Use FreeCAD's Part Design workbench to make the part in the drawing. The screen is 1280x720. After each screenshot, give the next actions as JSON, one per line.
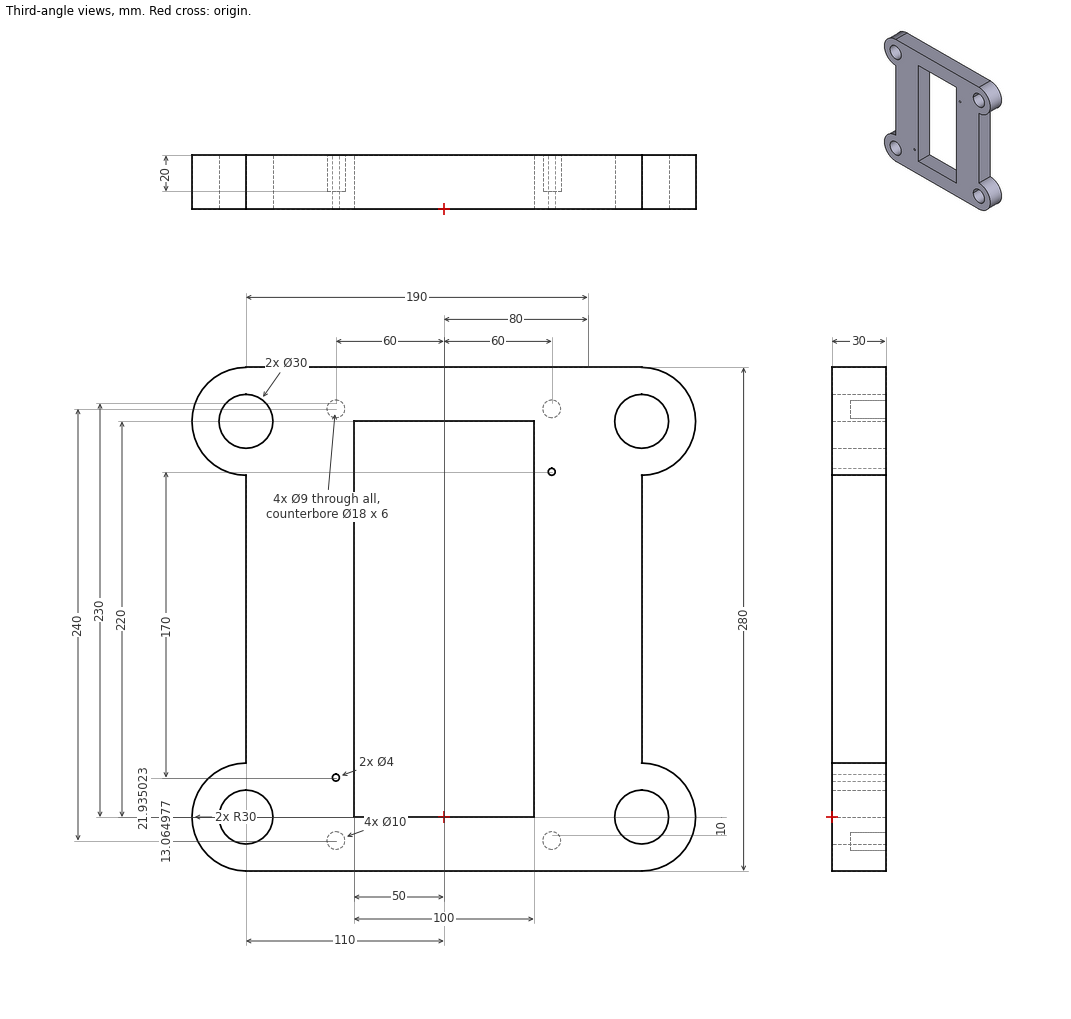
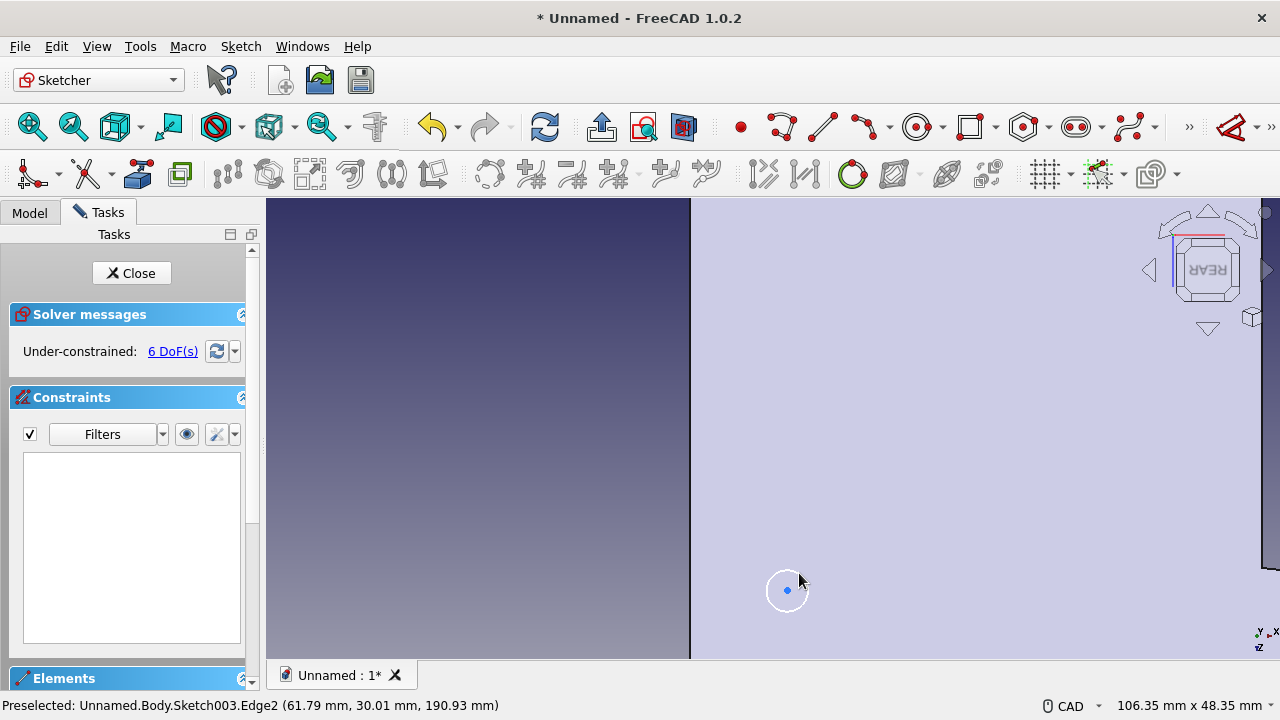
{"action": "scroll", "coordinate": [802, 577], "scroll_direction": "down", "scroll_amount": 9}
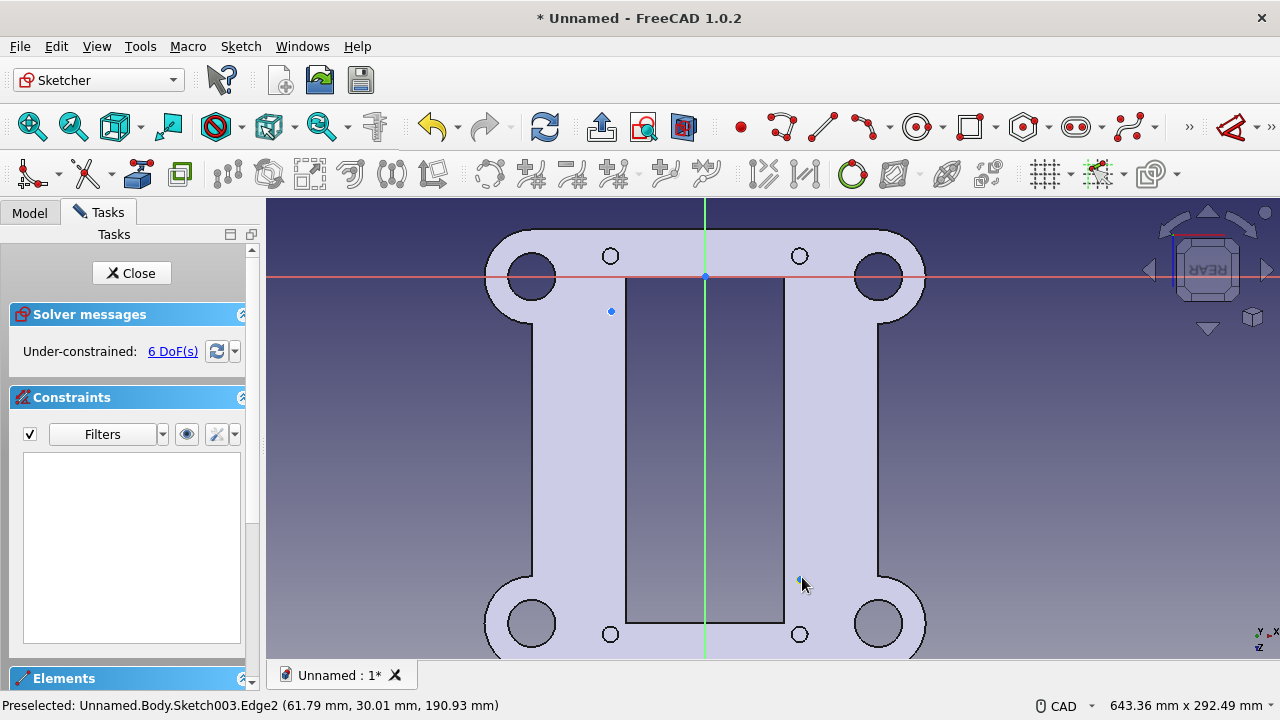
{"action": "scroll", "coordinate": [613, 310], "scroll_direction": "up", "scroll_amount": 8}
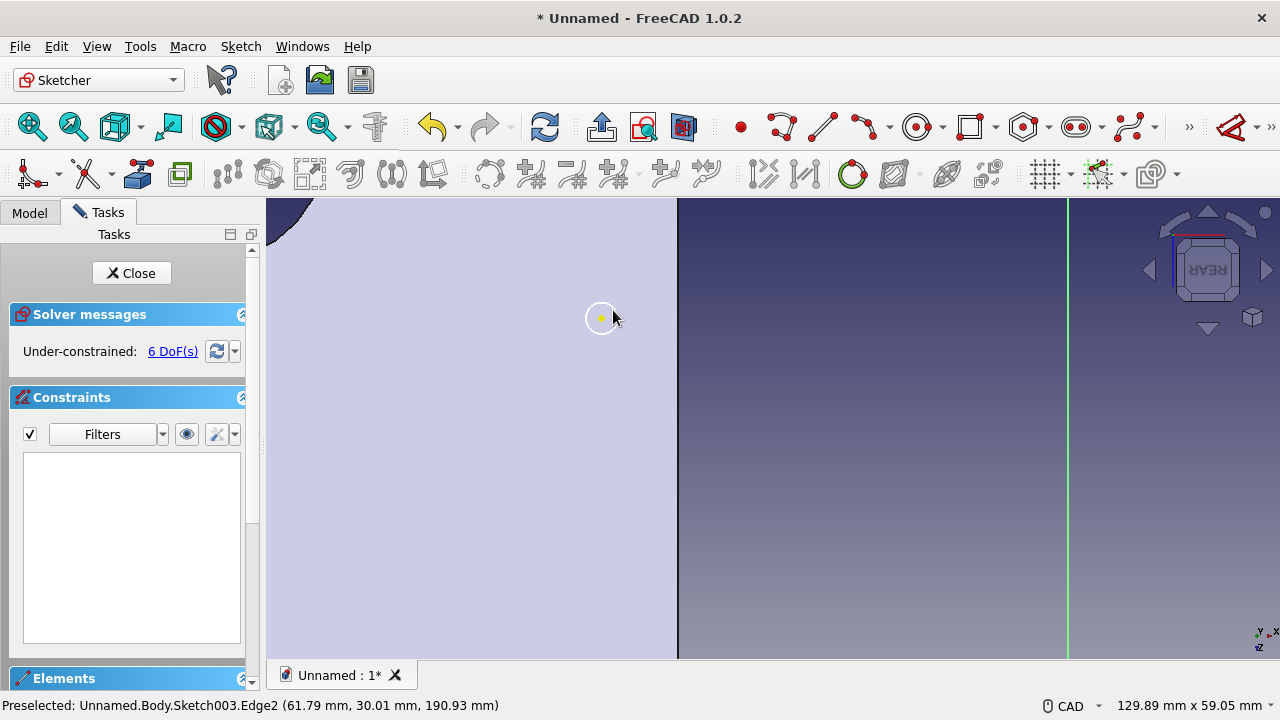
{"action": "left_click", "coordinate": [613, 307]}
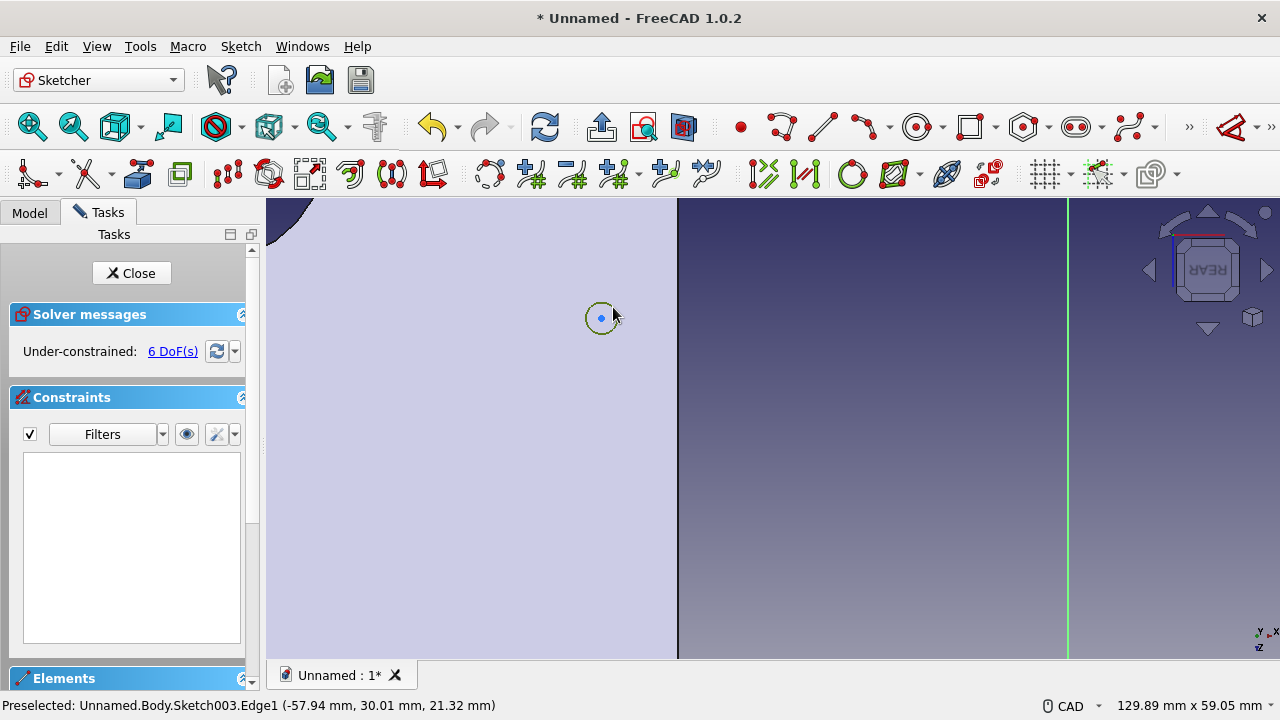
{"action": "scroll", "coordinate": [613, 309], "scroll_direction": "down", "scroll_amount": 8}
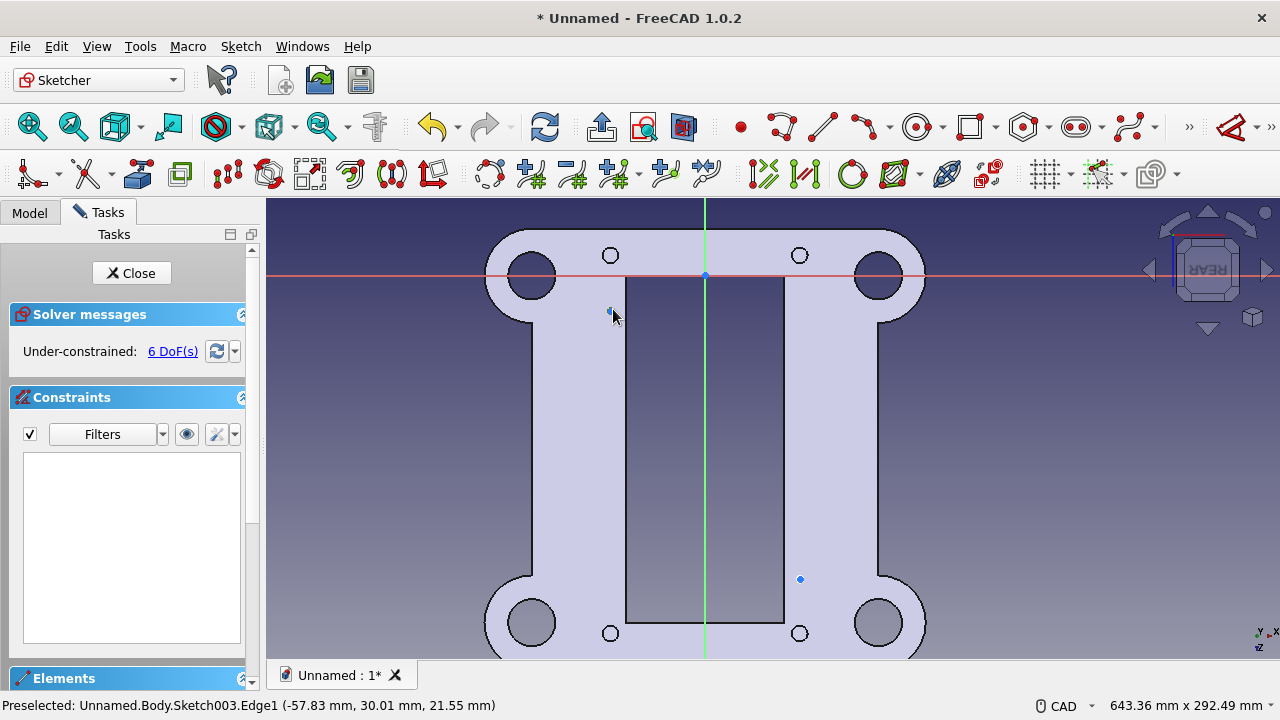
{"action": "scroll", "coordinate": [802, 577], "scroll_direction": "up", "scroll_amount": 7}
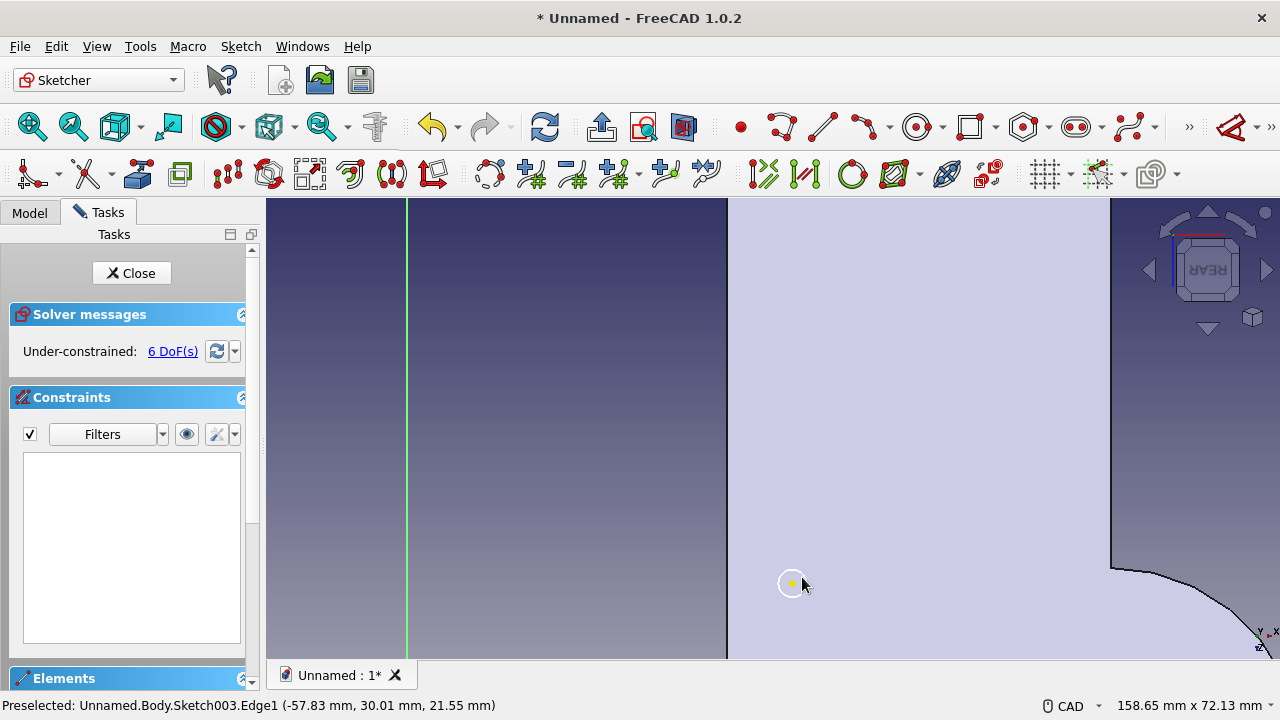
{"action": "left_click", "coordinate": [802, 574]}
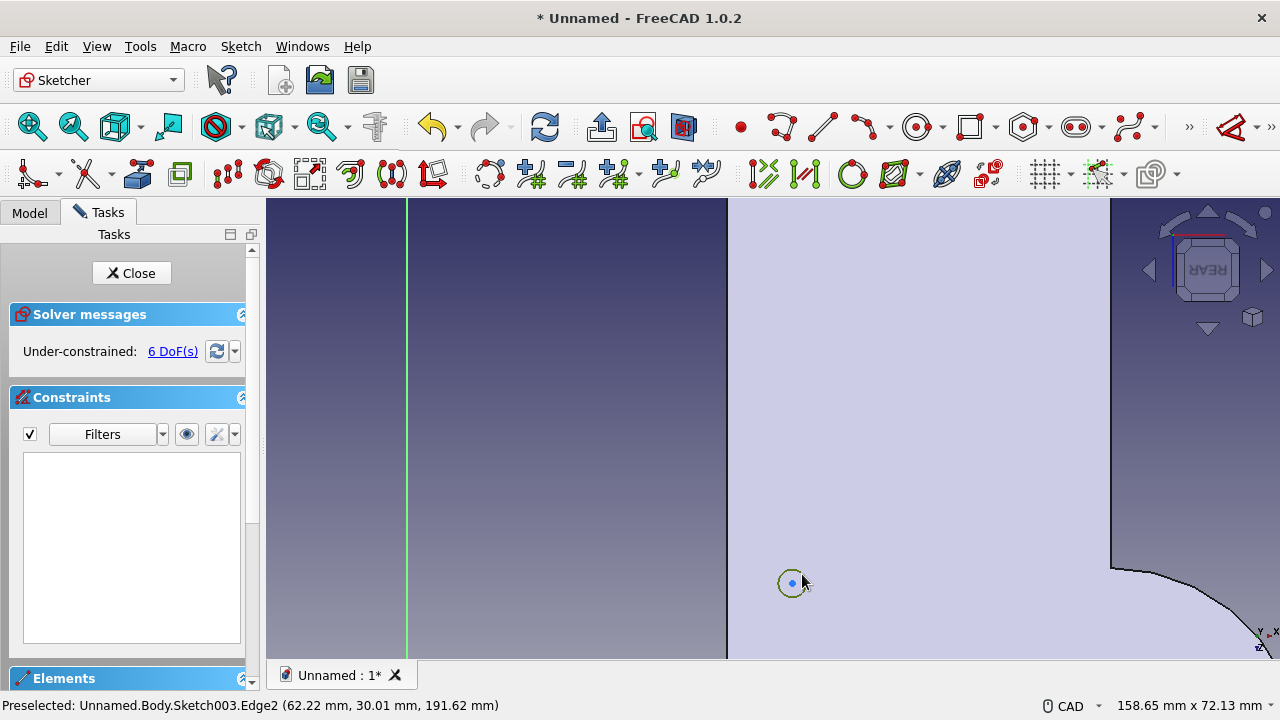
{"action": "key", "text": "e"}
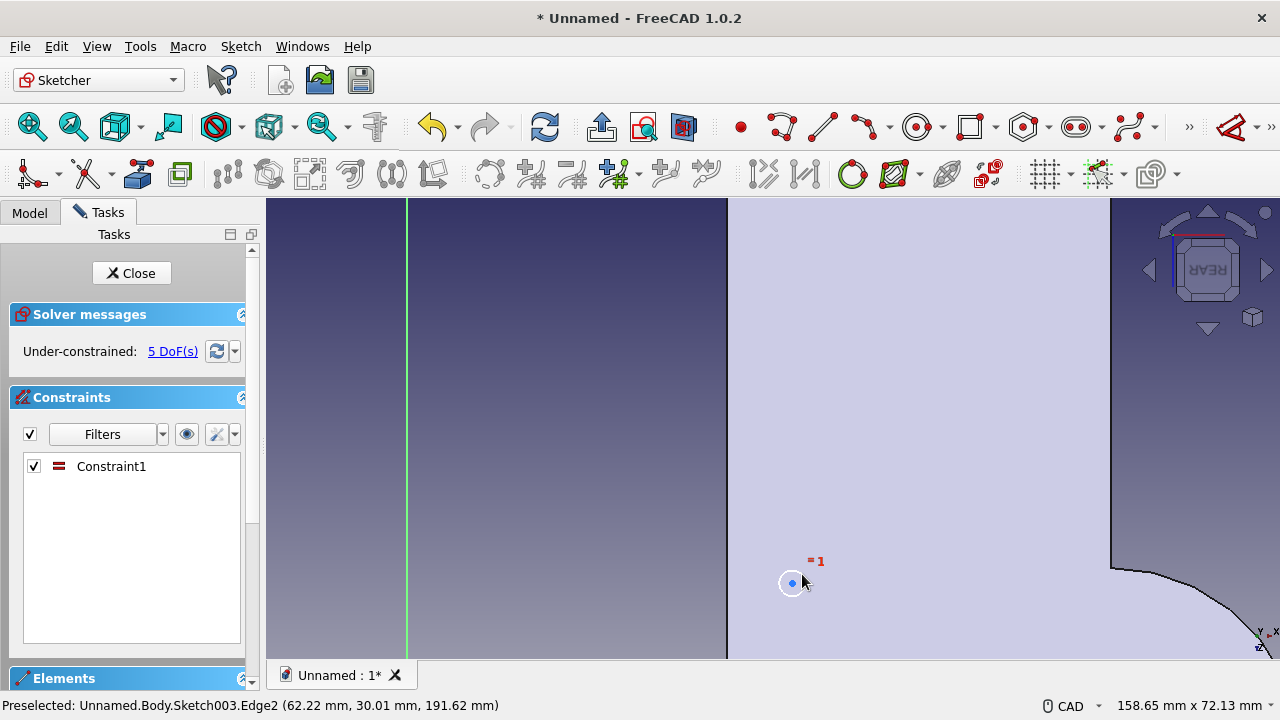
{"action": "left_click", "coordinate": [1230, 128]}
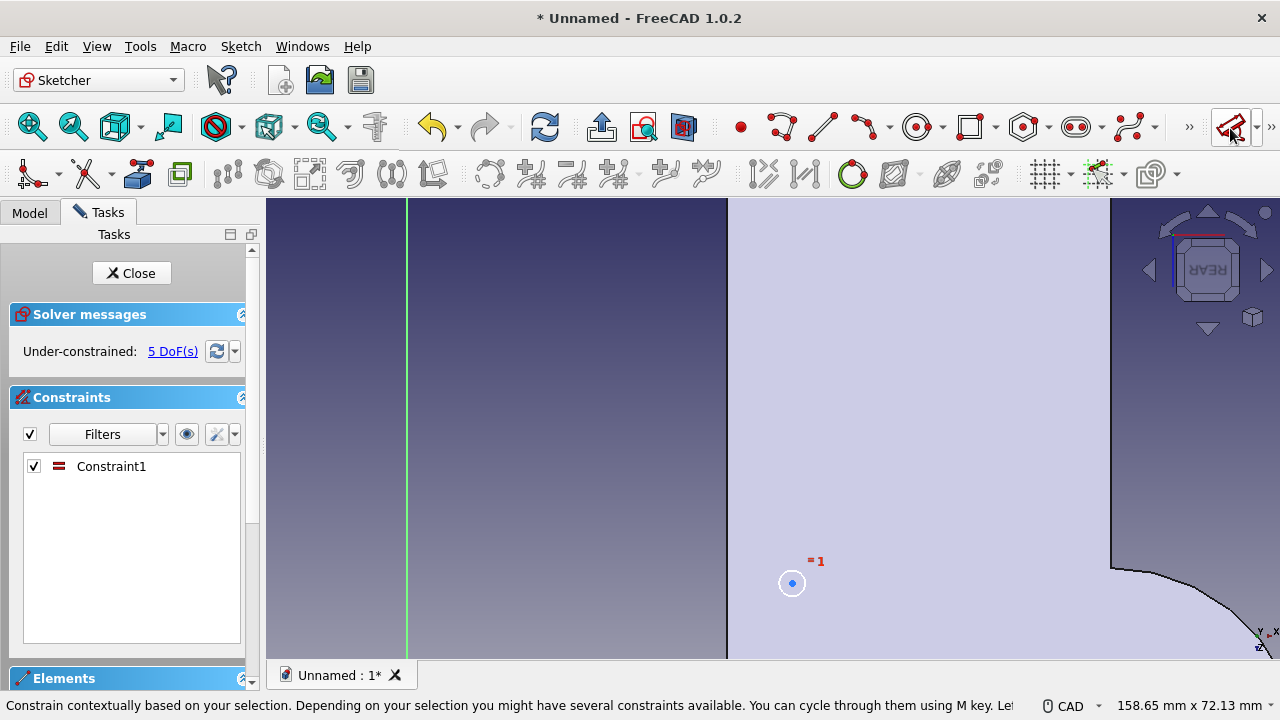
{"action": "scroll", "coordinate": [802, 577], "scroll_direction": "down", "scroll_amount": 7}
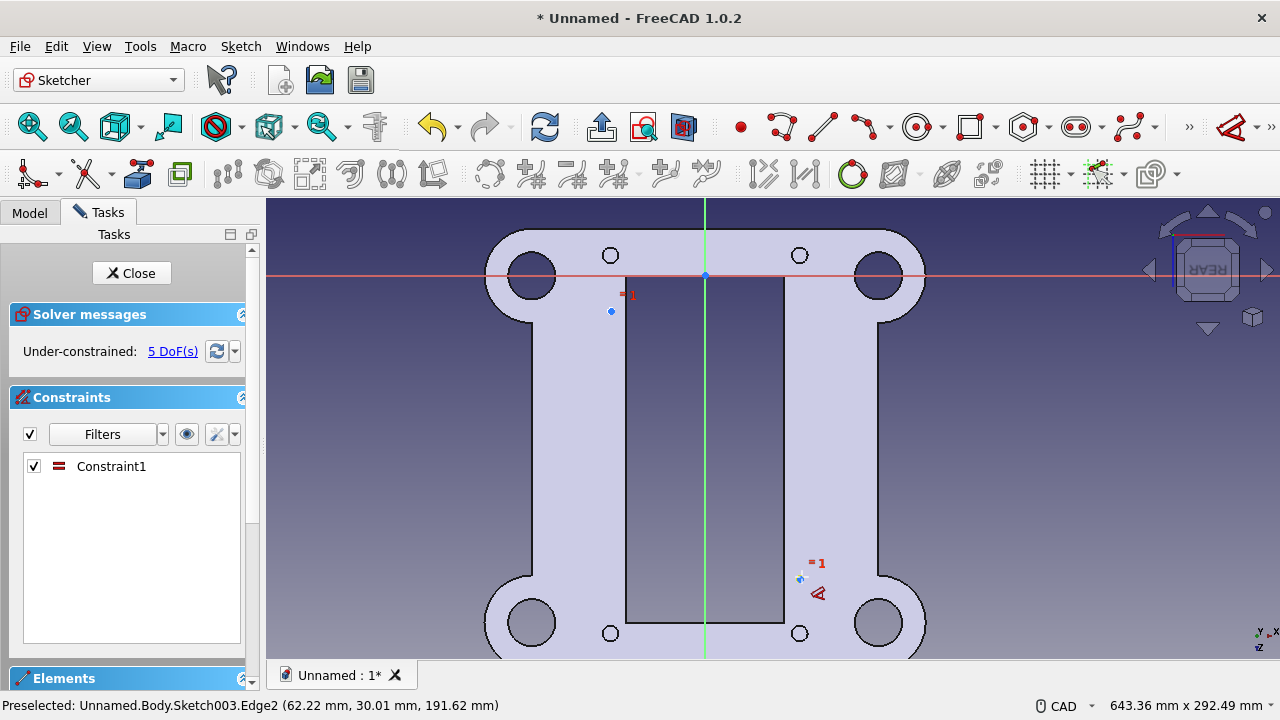
{"action": "scroll", "coordinate": [613, 309], "scroll_direction": "up", "scroll_amount": 10}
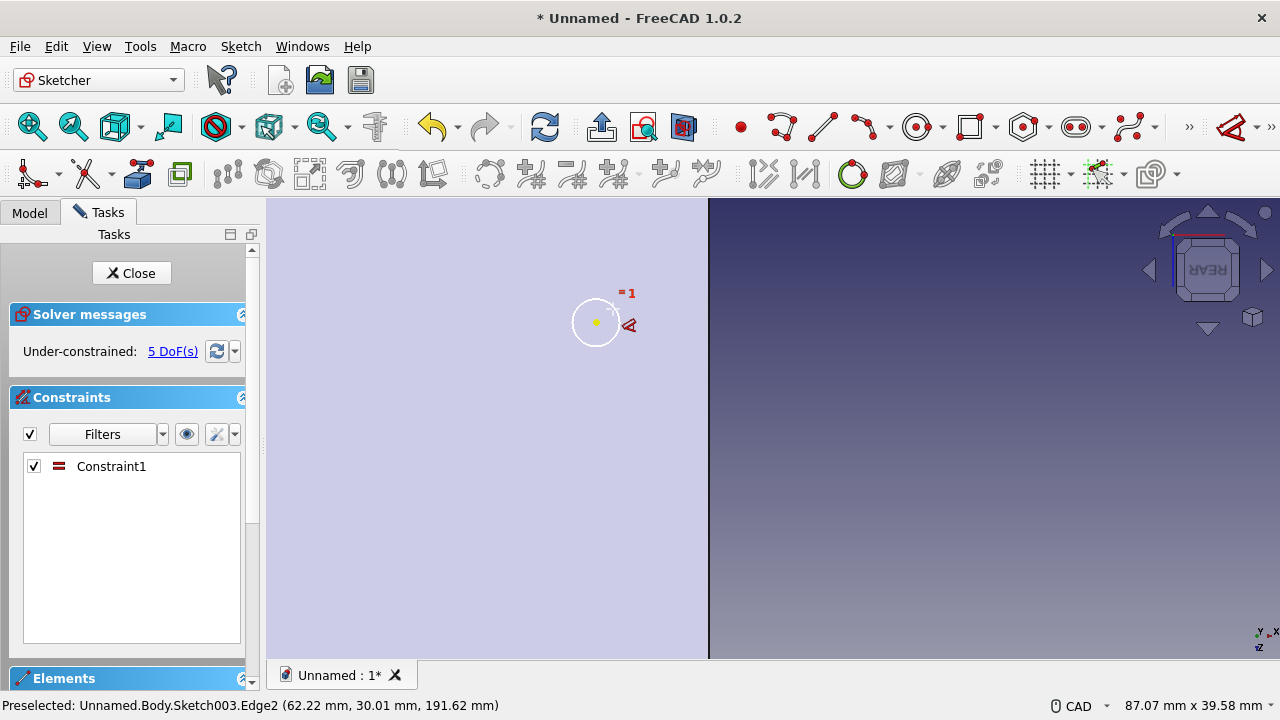
{"action": "left_click", "coordinate": [613, 306]}
{"action": "left_click", "coordinate": [636, 284]}